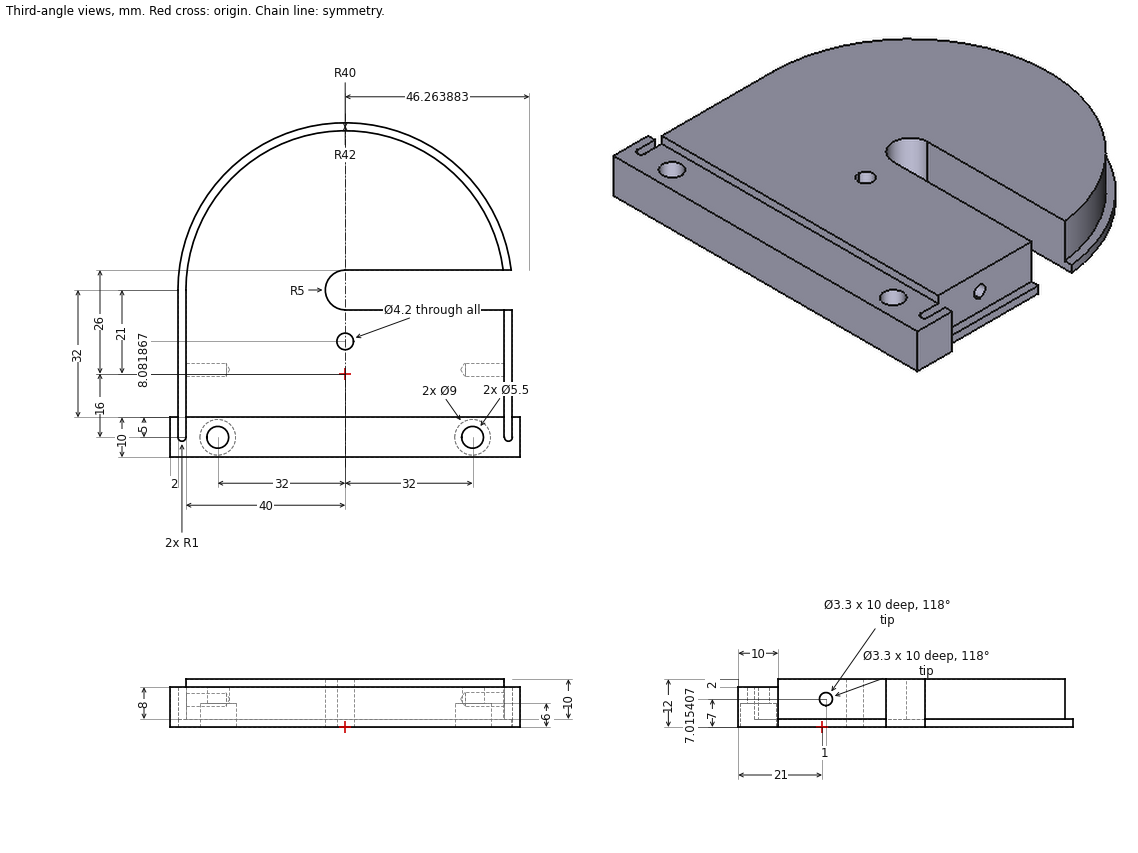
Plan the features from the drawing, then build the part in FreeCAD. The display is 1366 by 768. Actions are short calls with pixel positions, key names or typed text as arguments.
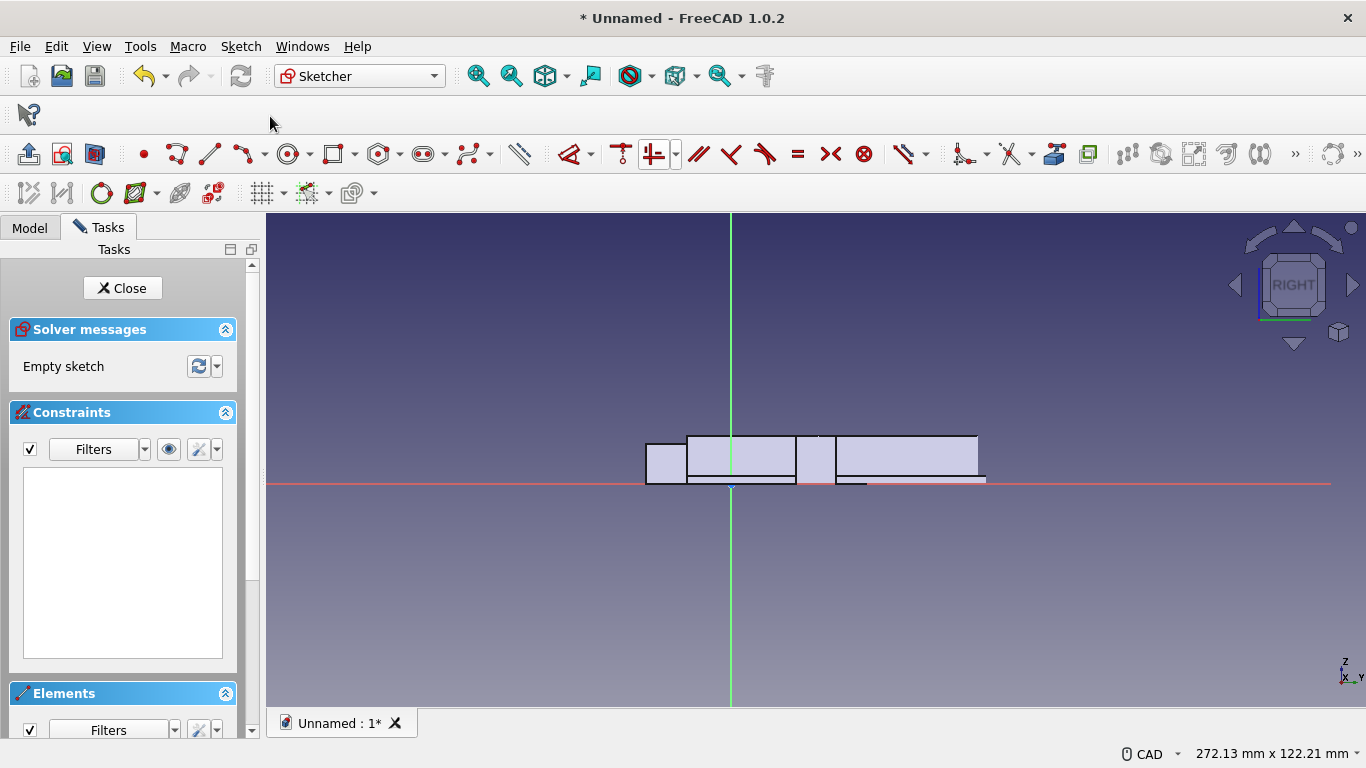
key(q)
key(s)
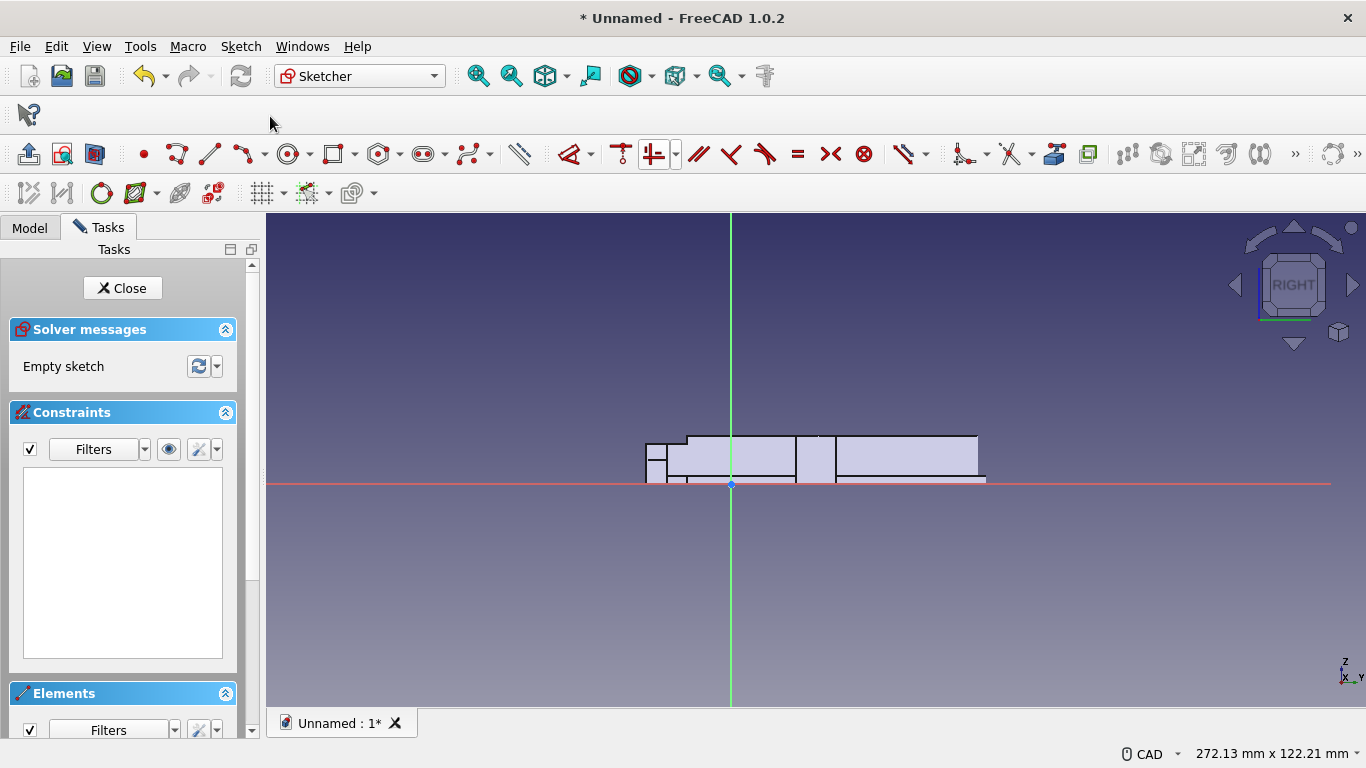
scroll(735, 456, up, 15)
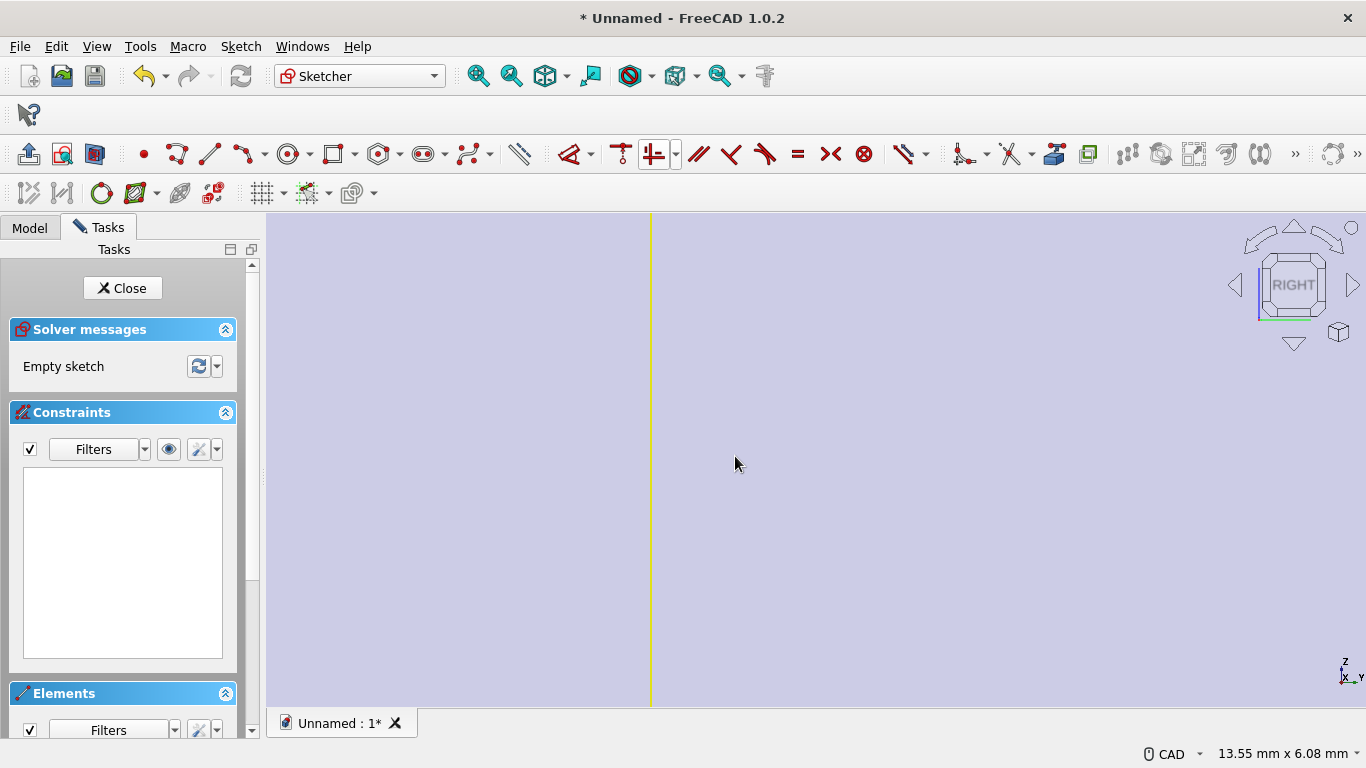
key(g)
key(c)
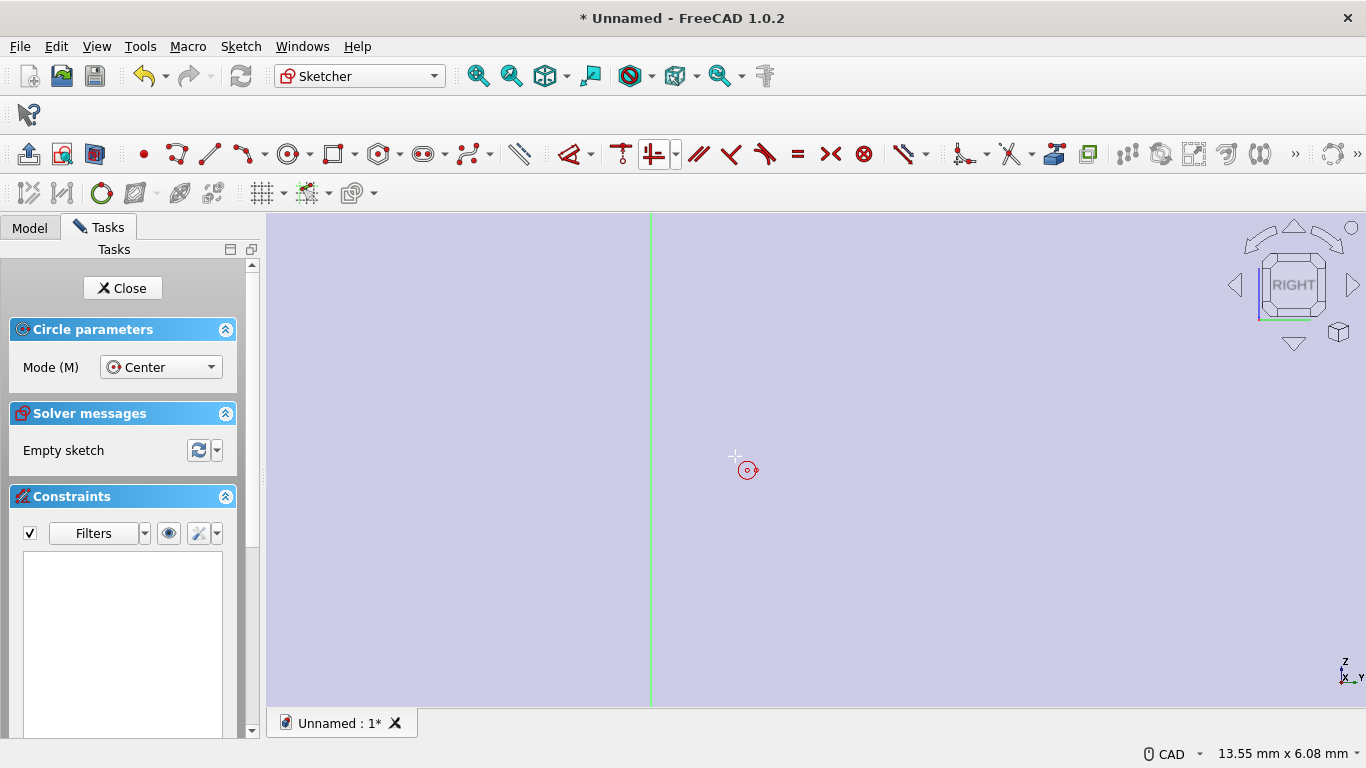
click(732, 444)
click(827, 350)
key(Escape)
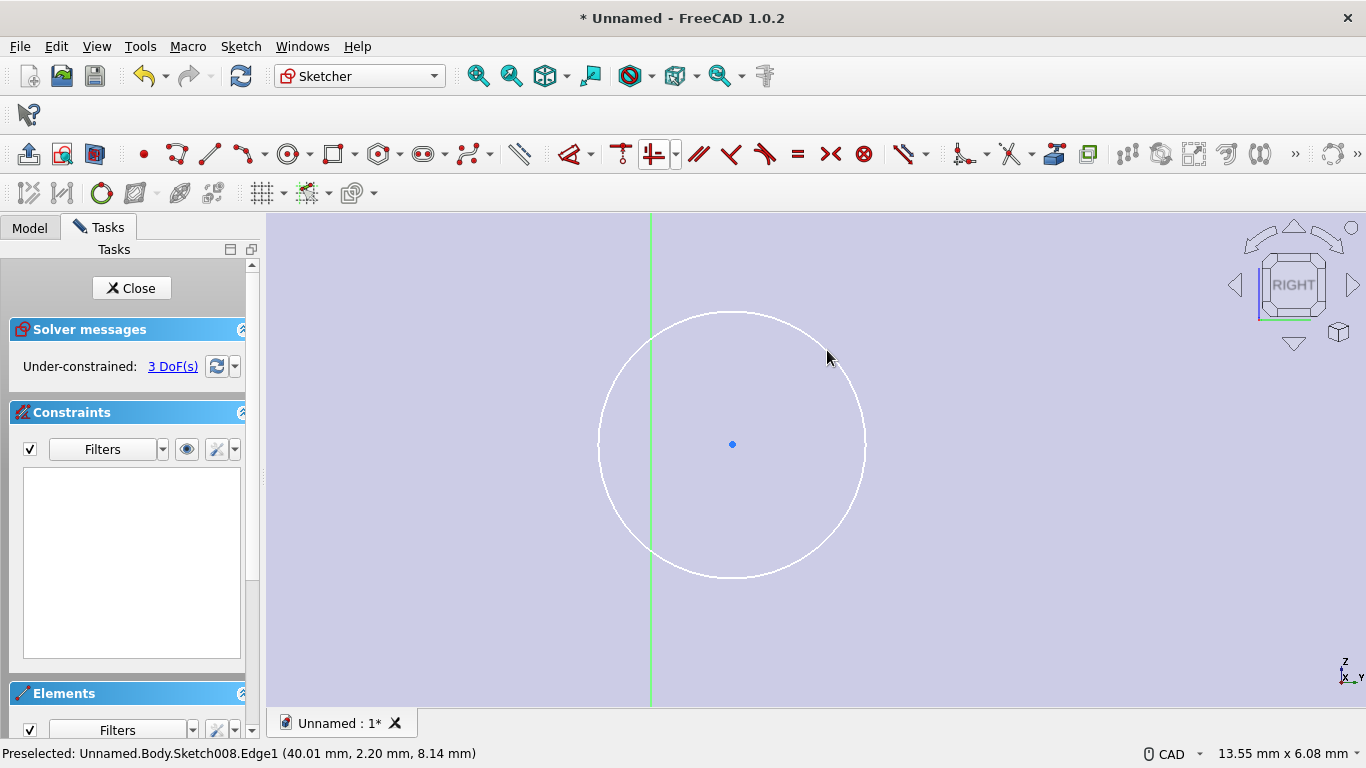
click(568, 154)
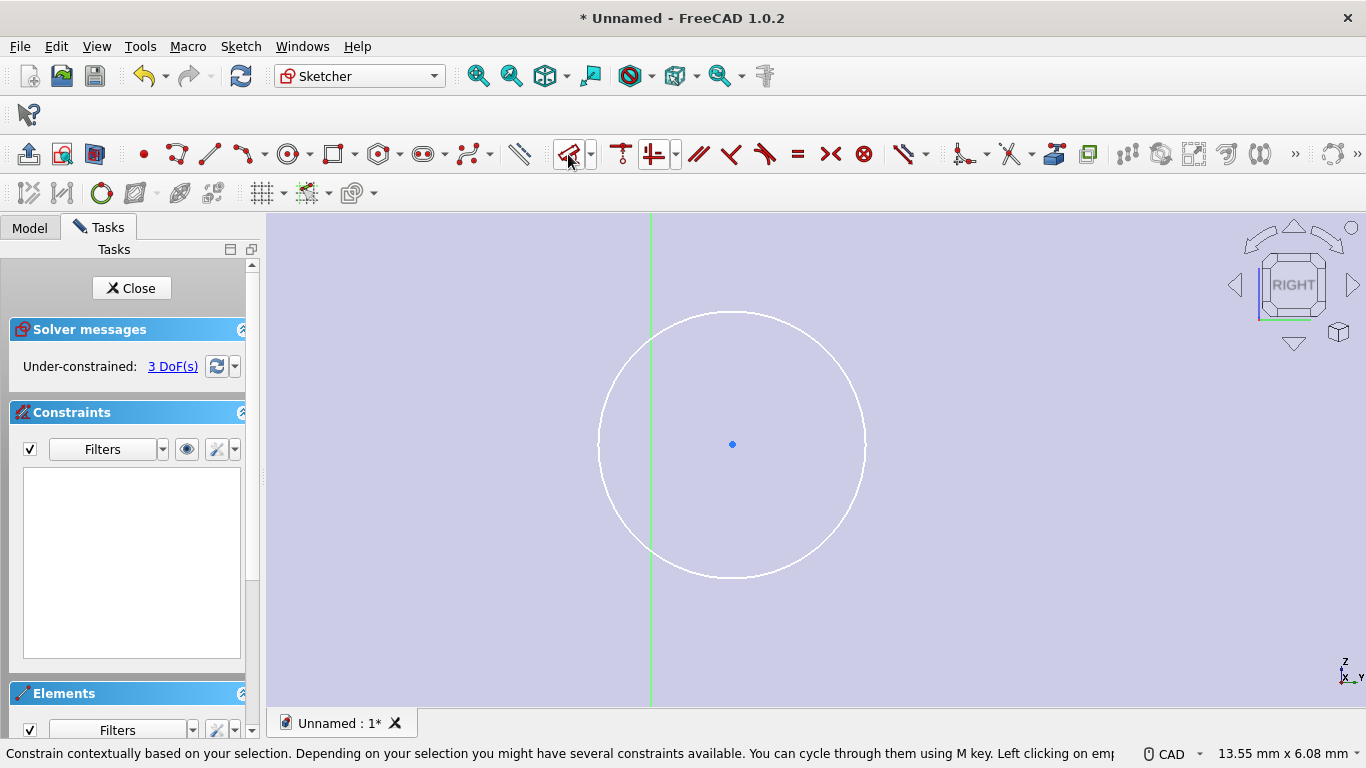
click(826, 350)
click(849, 327)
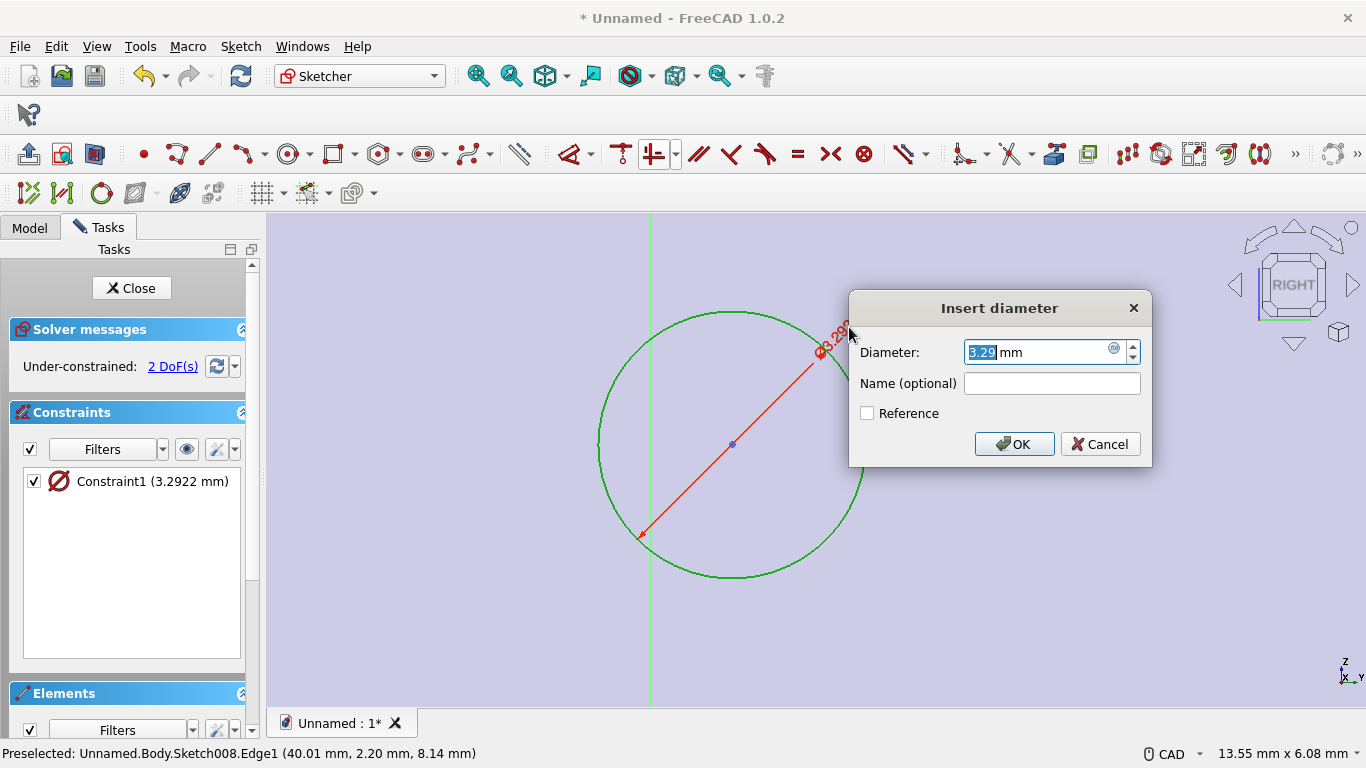
text(3.3)
key(Return)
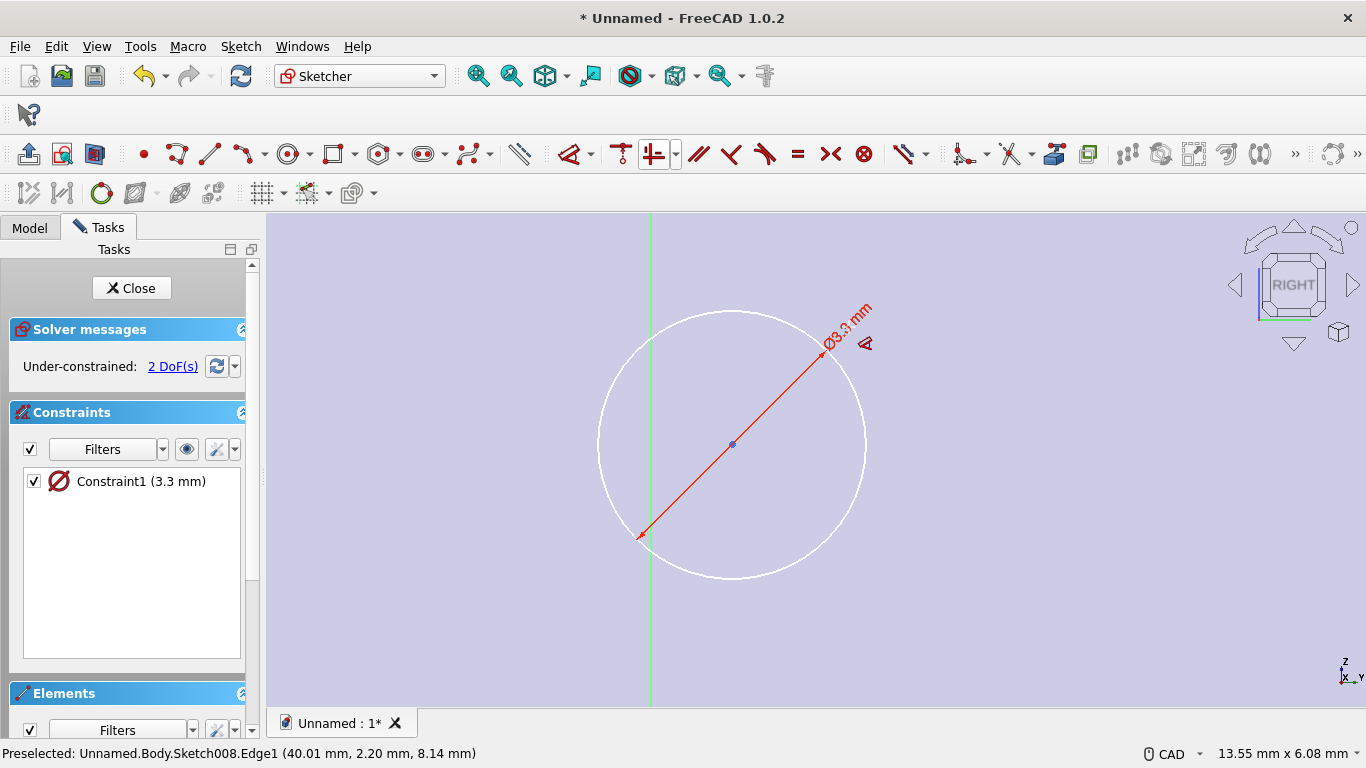
click(732, 445)
click(691, 411)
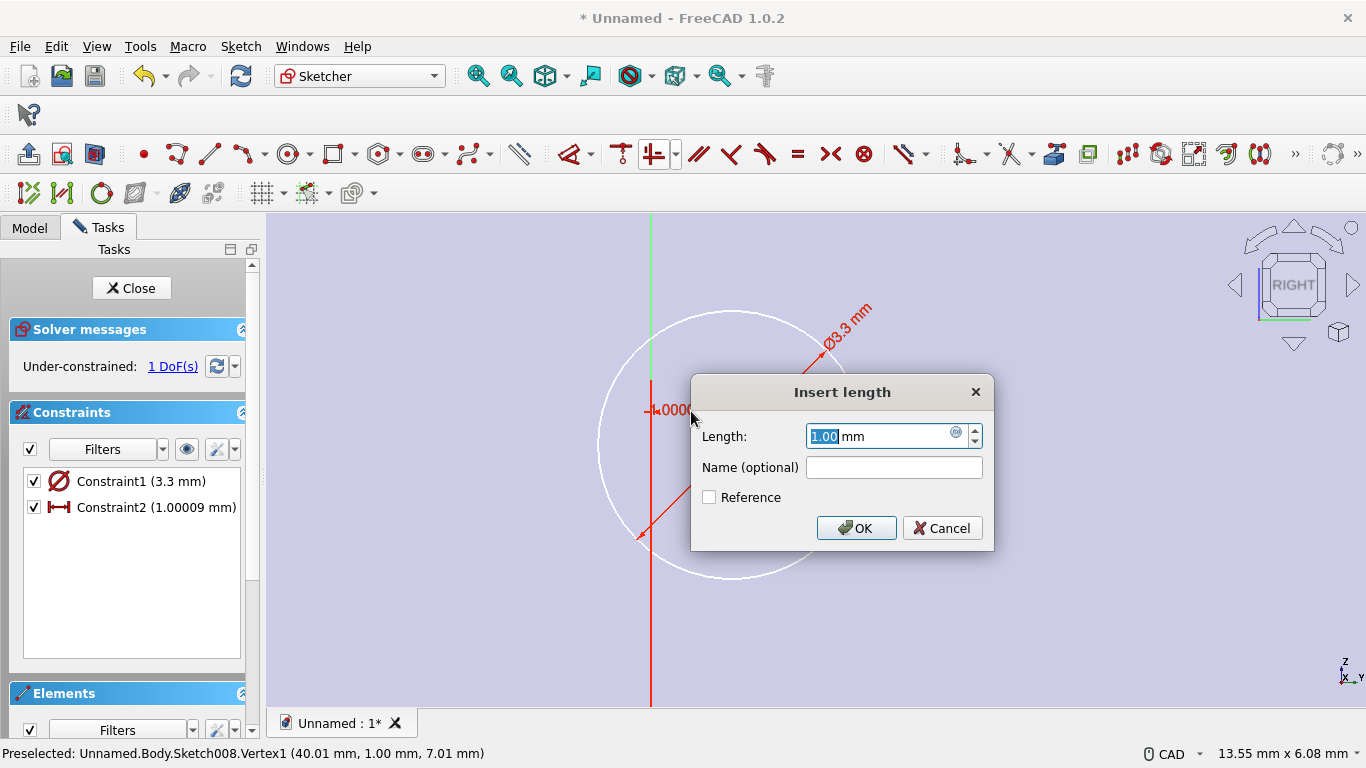
text(1)
key(Return)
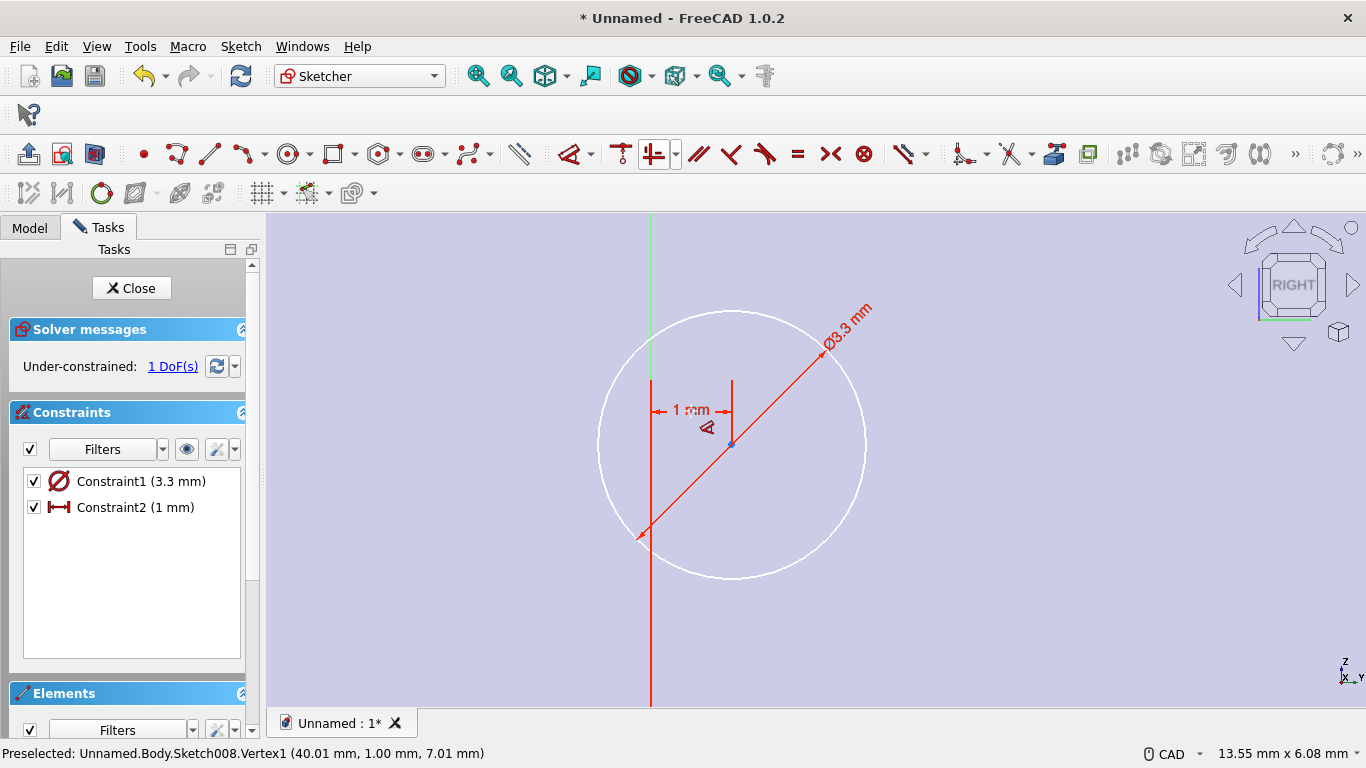
click(732, 445)
click(617, 562)